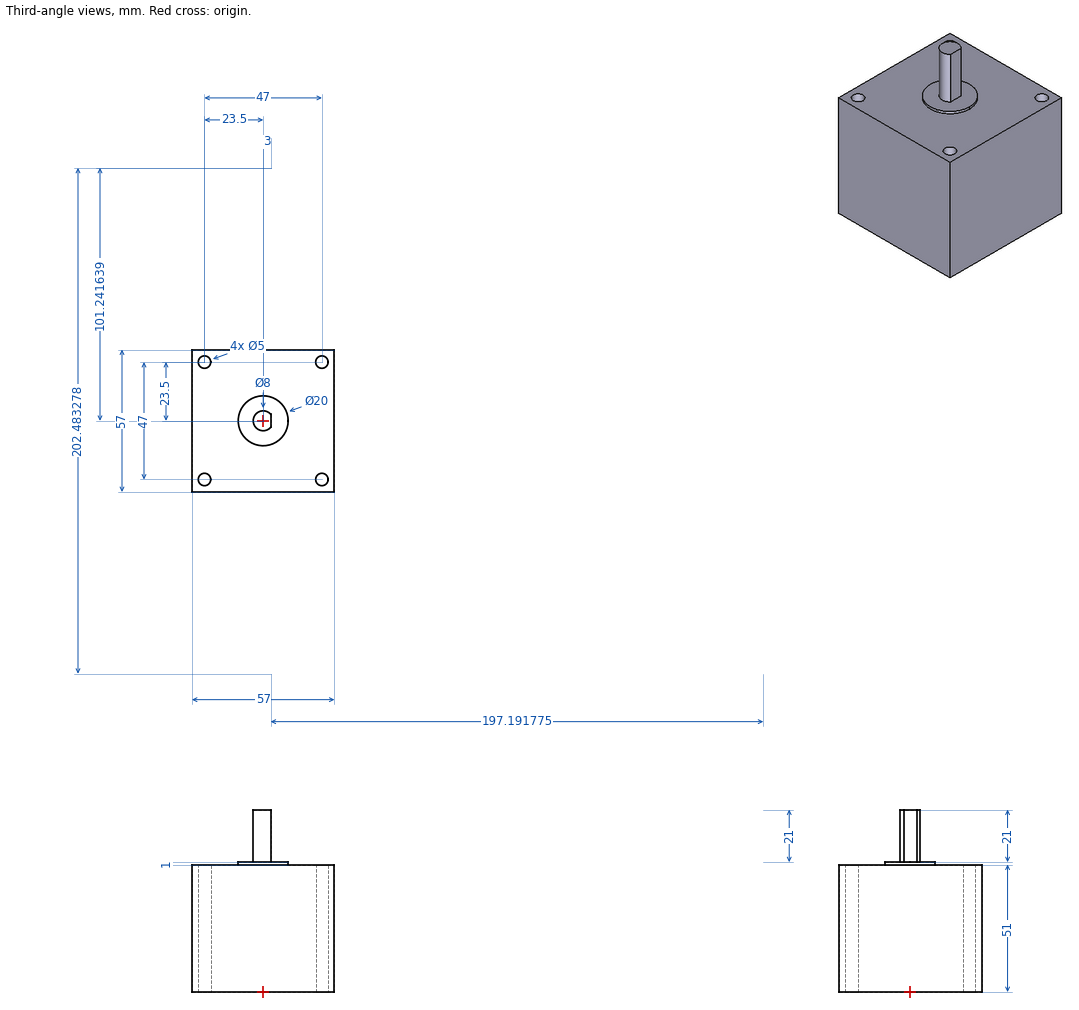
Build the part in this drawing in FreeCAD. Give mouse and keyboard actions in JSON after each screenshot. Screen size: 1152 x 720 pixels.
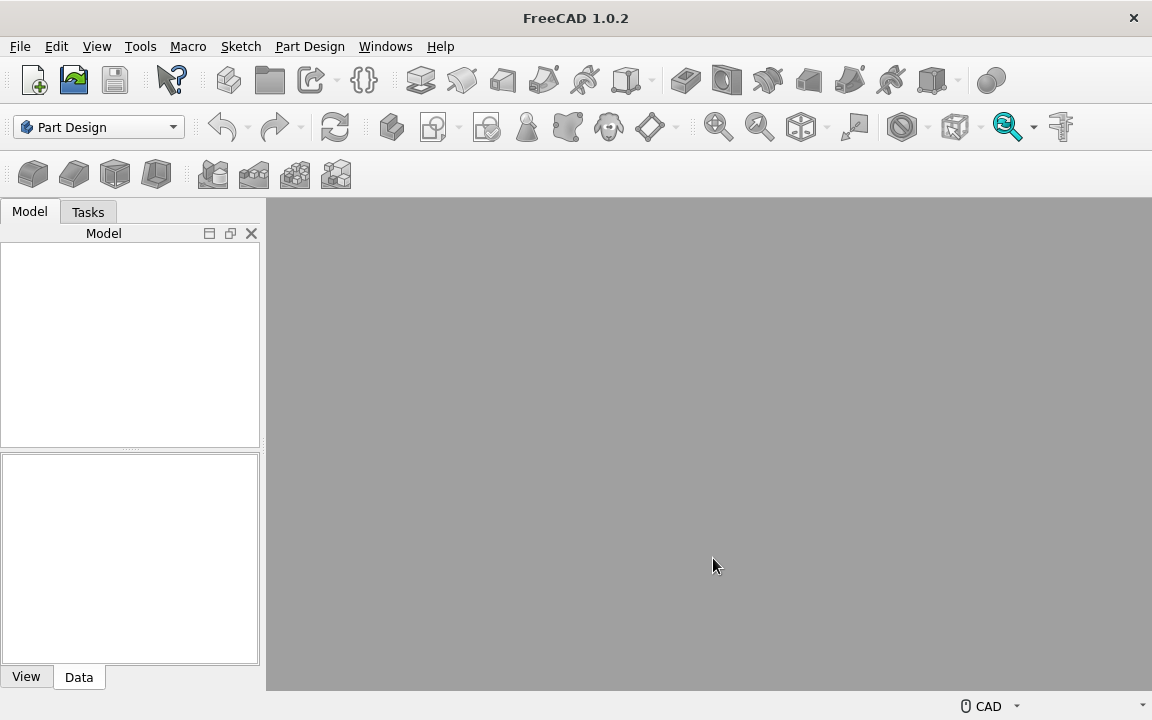
{"action": "left_click", "coordinate": [33, 80]}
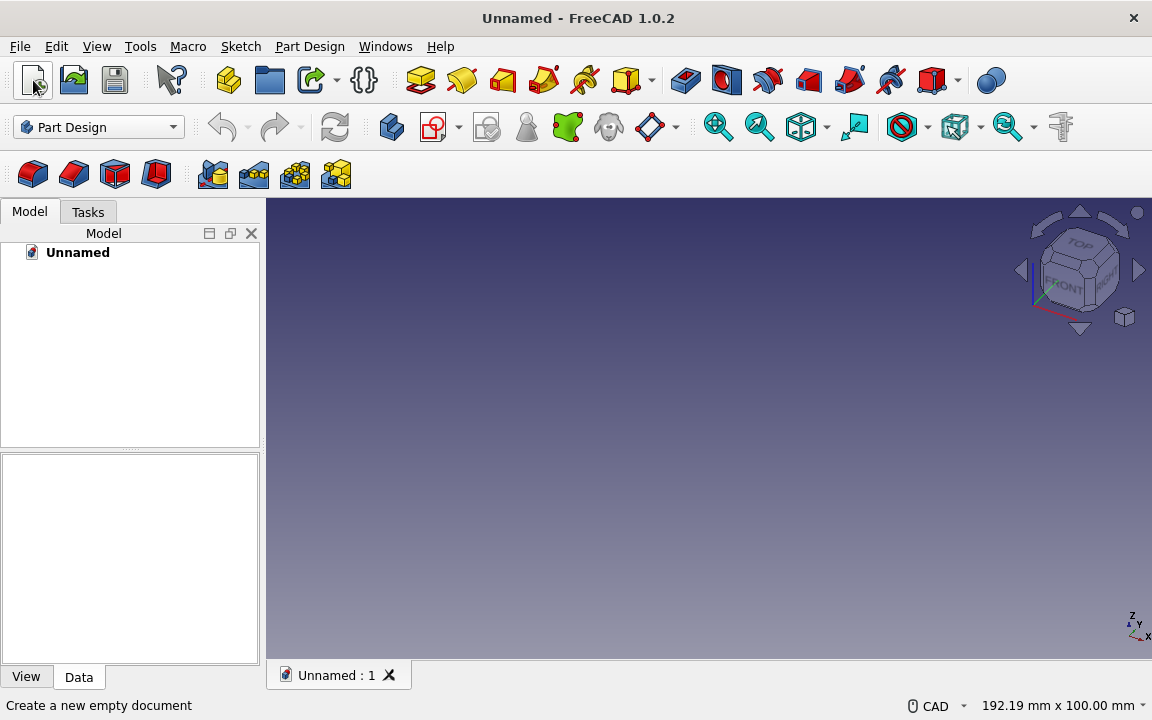
{"action": "left_click", "coordinate": [432, 128]}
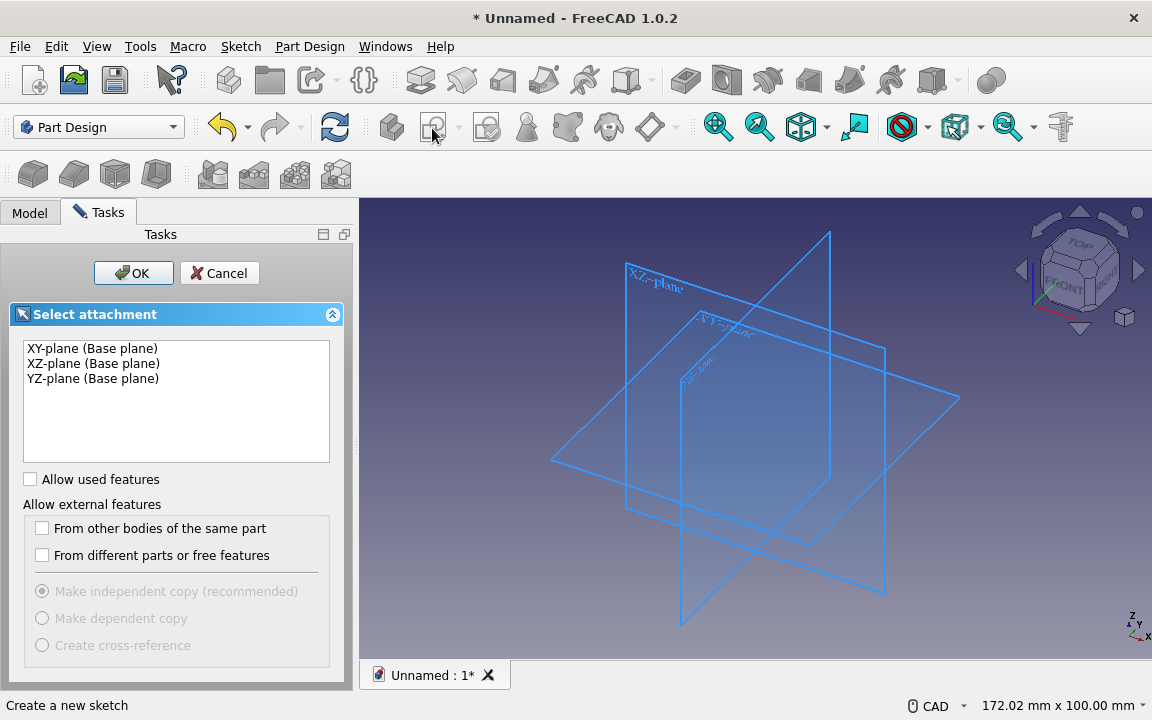
{"action": "left_click", "coordinate": [84, 348]}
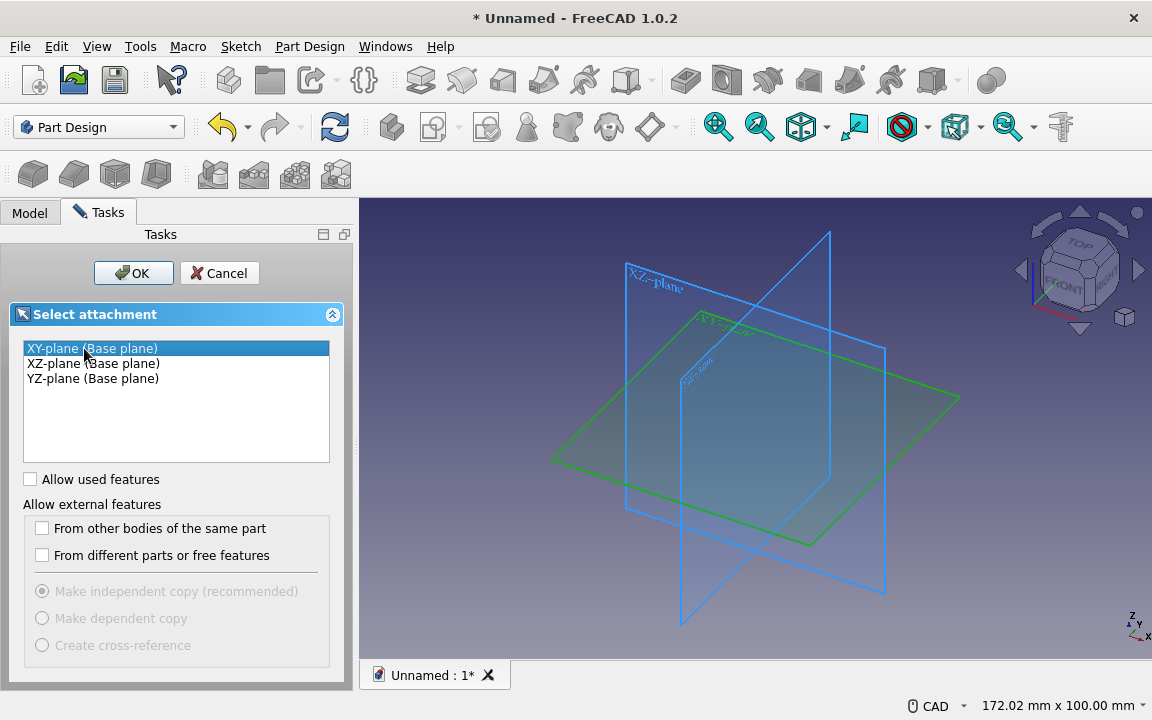
{"action": "left_click", "coordinate": [134, 273]}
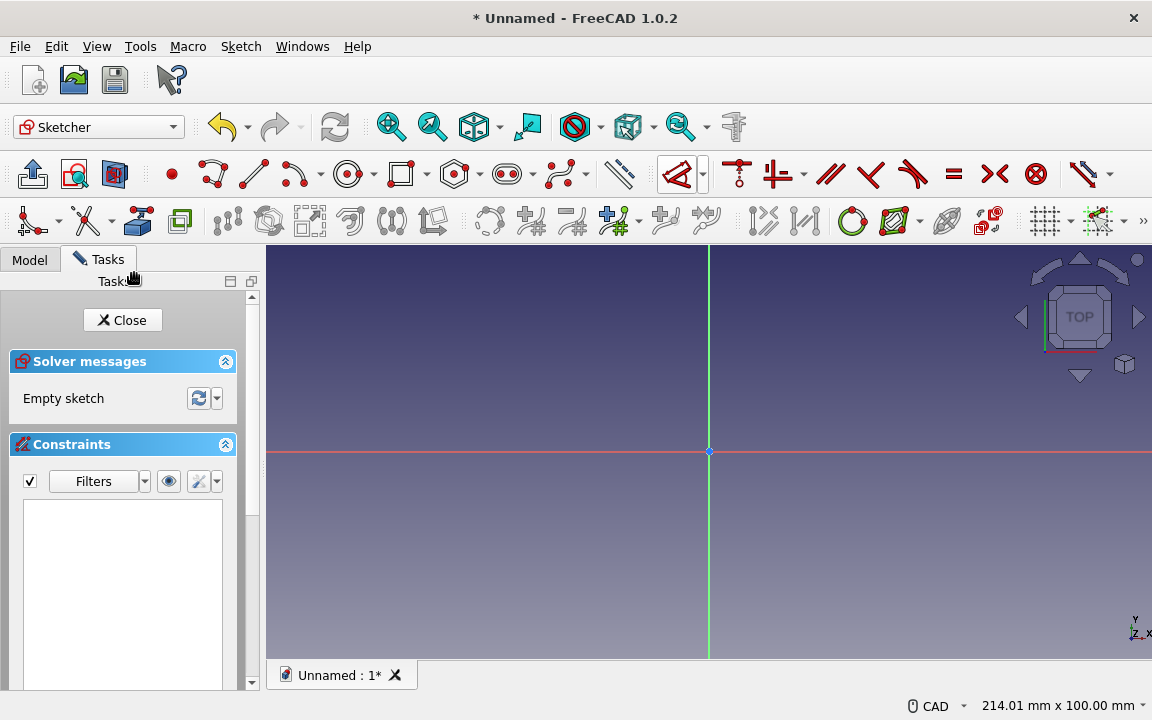
{"action": "left_click", "coordinate": [426, 174]}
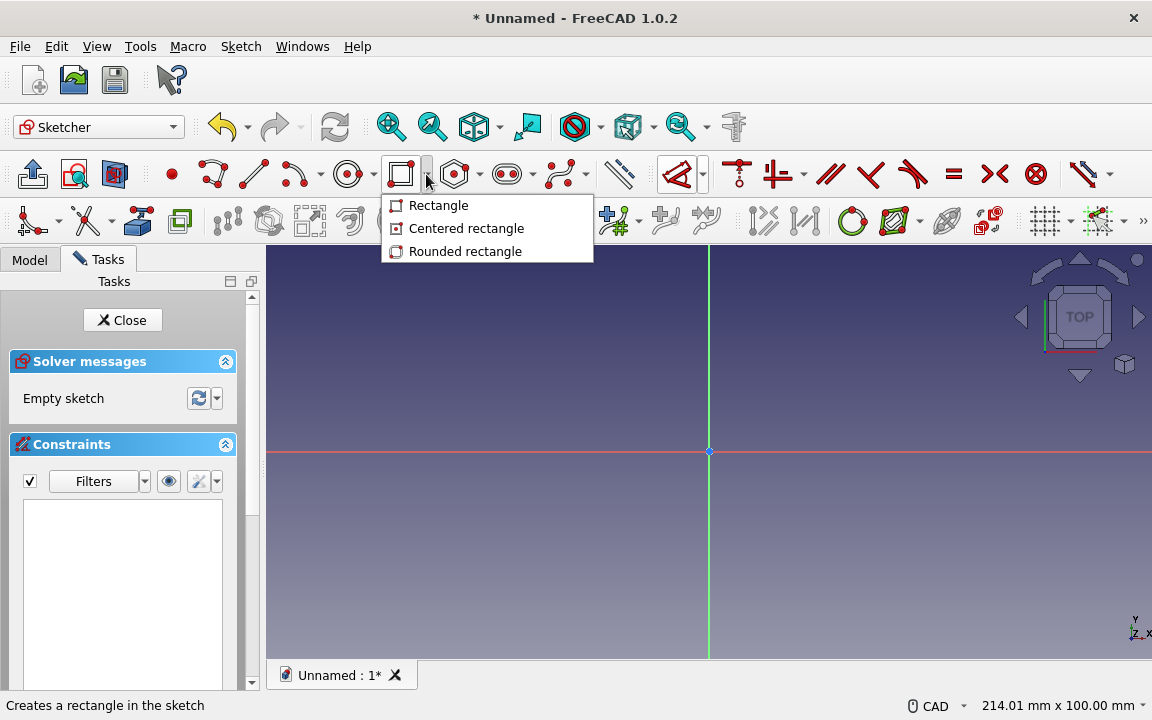
{"action": "left_click", "coordinate": [488, 228]}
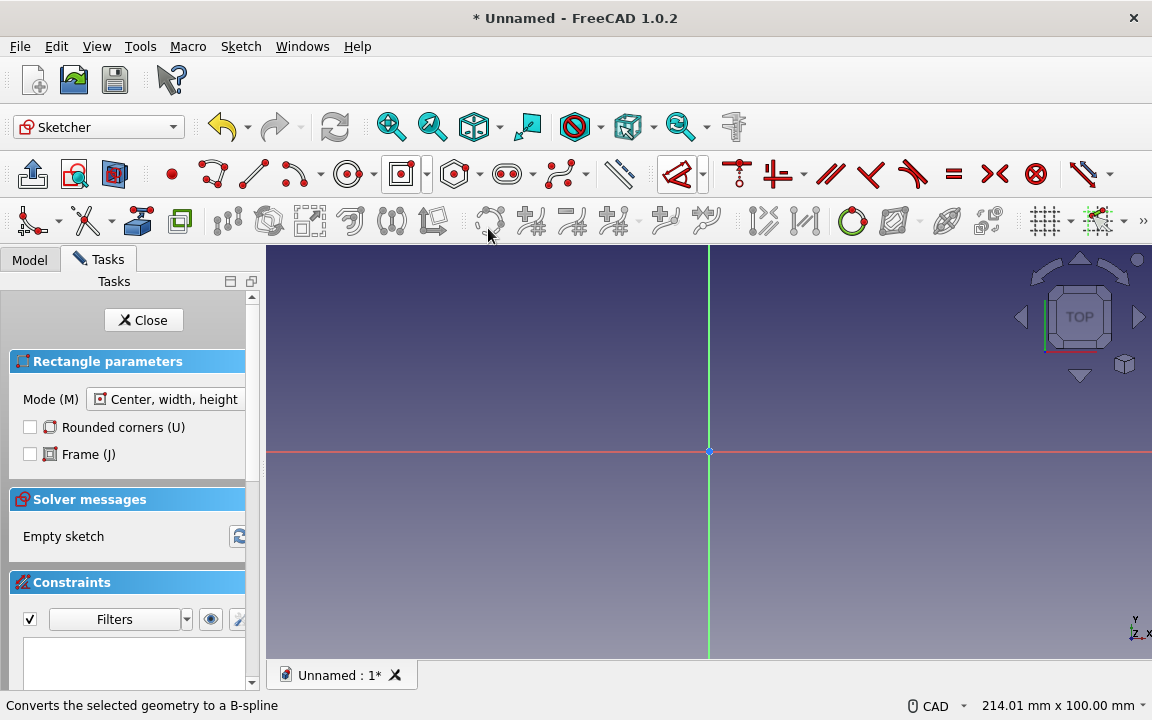
{"action": "left_click", "coordinate": [709, 452]}
{"action": "left_click", "coordinate": [827, 334]}
{"action": "key", "text": "Escape"}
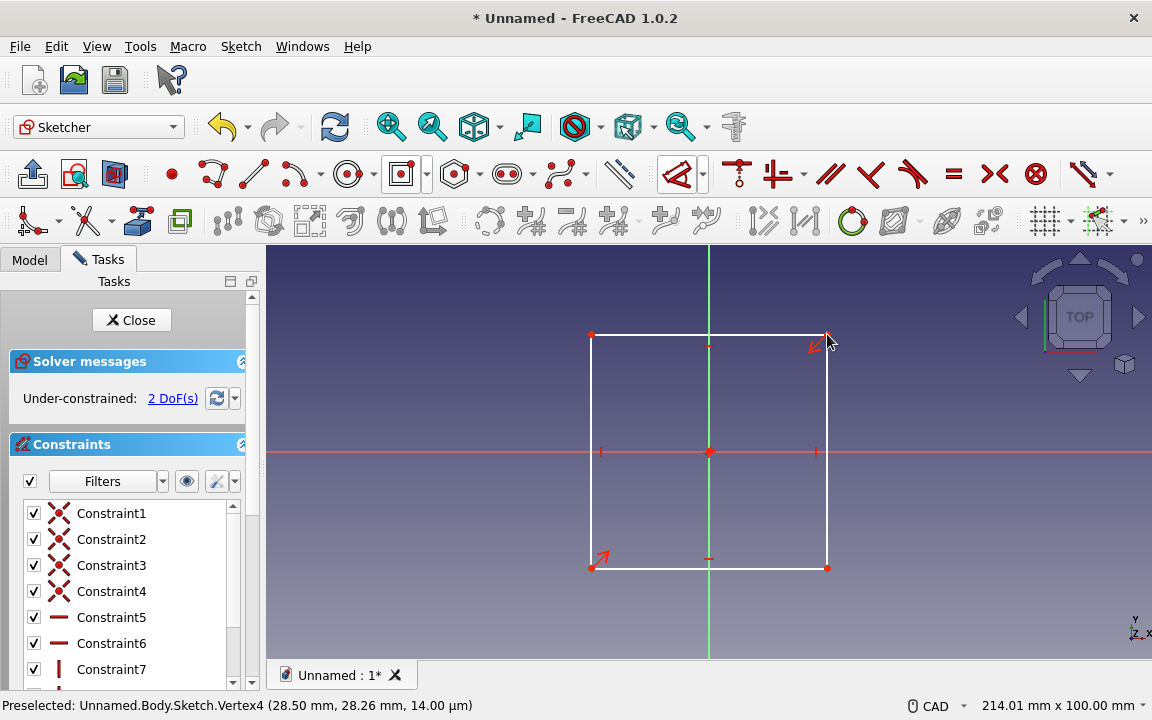
{"action": "left_click", "coordinate": [676, 174]}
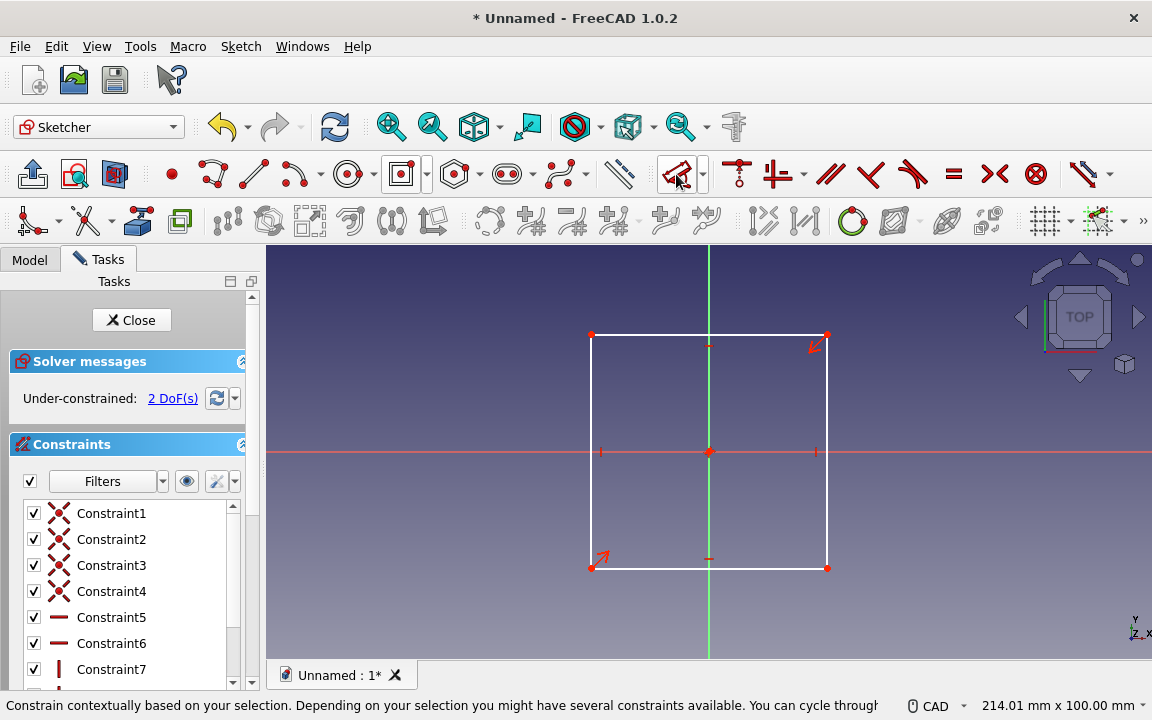
{"action": "left_click", "coordinate": [662, 569]}
{"action": "left_click", "coordinate": [655, 603]}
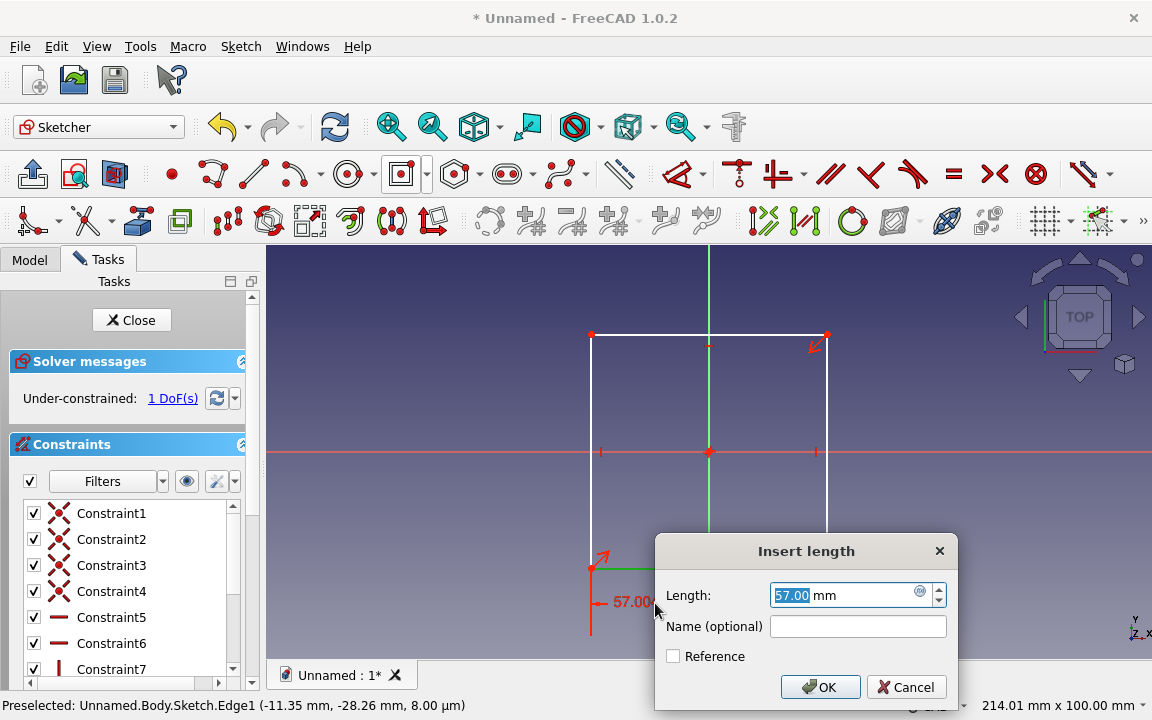
{"action": "type", "text": "57"}
{"action": "key", "text": "Return"}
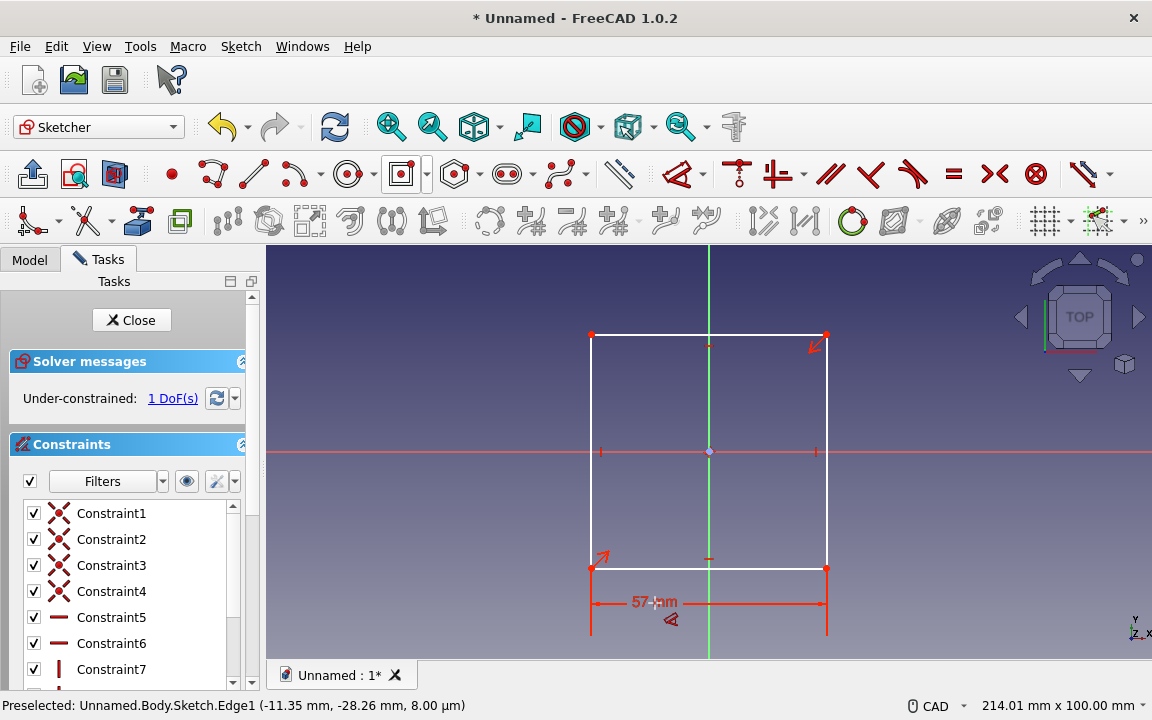
{"action": "left_click", "coordinate": [827, 499]}
{"action": "left_click", "coordinate": [861, 398]}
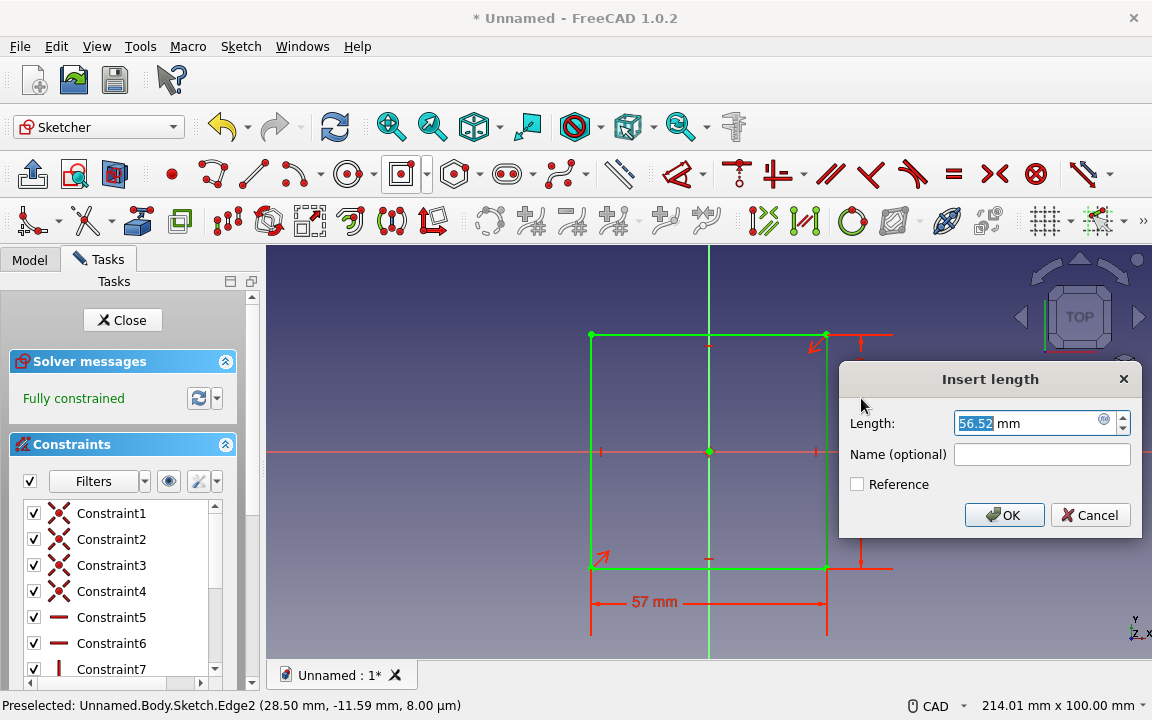
{"action": "type", "text": "57"}
{"action": "key", "text": "Return"}
{"action": "key", "text": "Escape"}